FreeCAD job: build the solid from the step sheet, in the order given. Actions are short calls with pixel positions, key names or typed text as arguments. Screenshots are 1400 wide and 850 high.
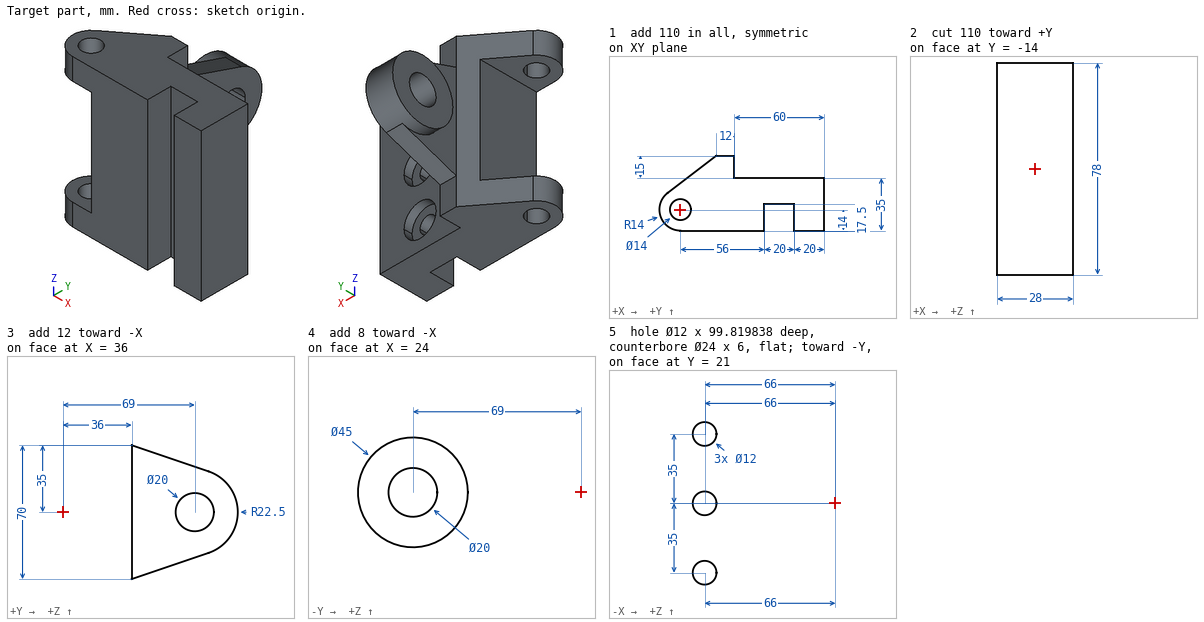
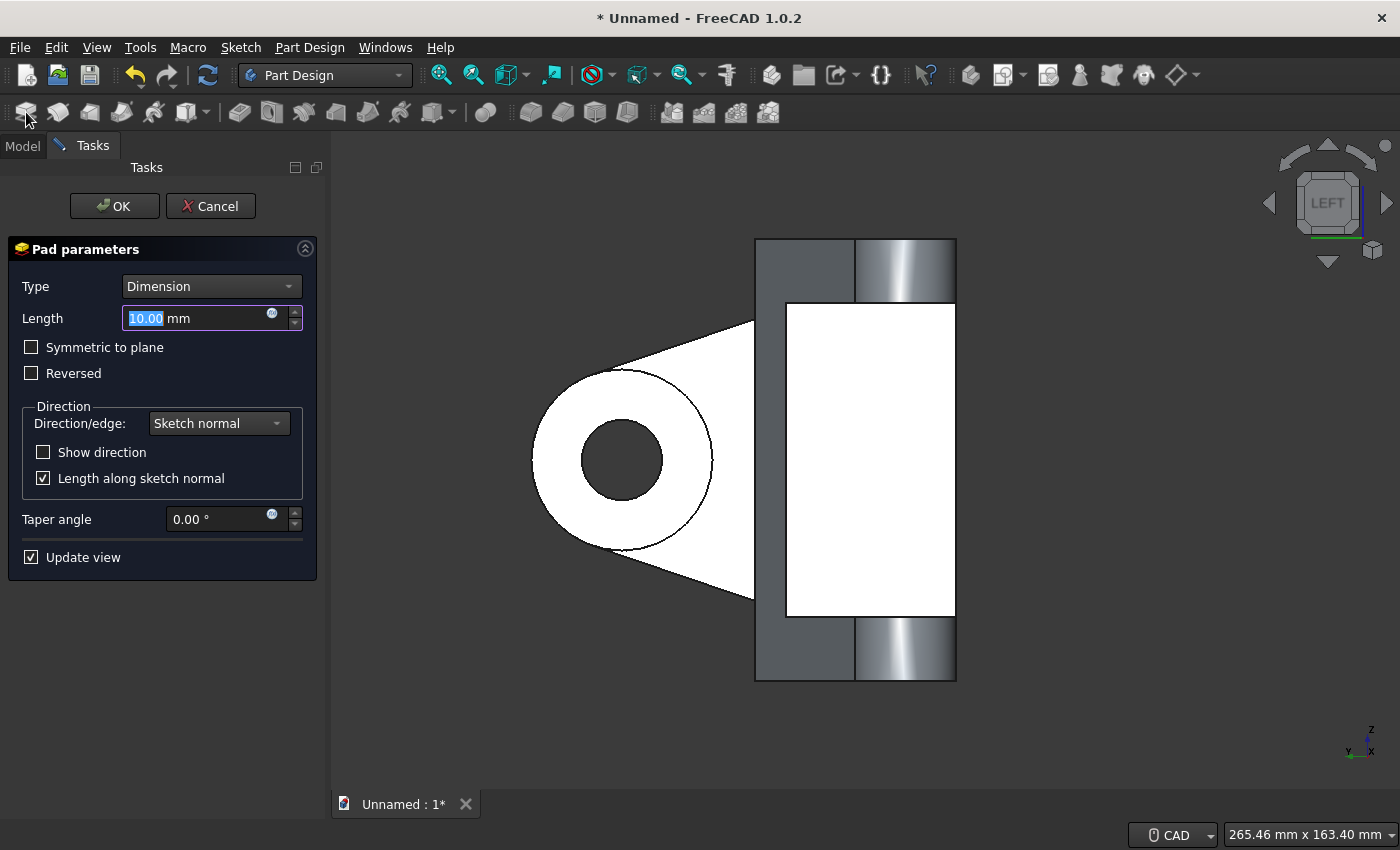
text(8)
key(Tab)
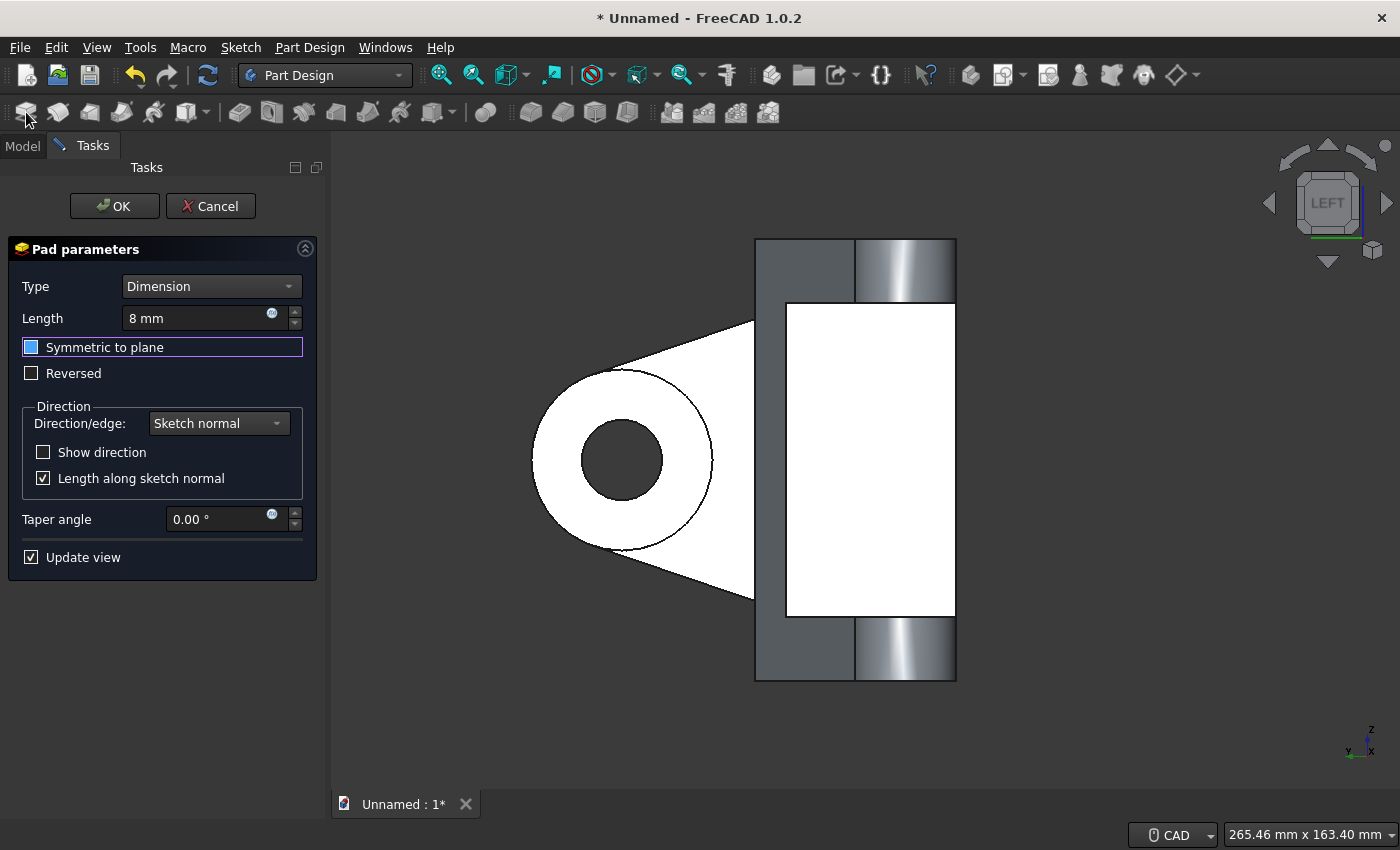
click(115, 206)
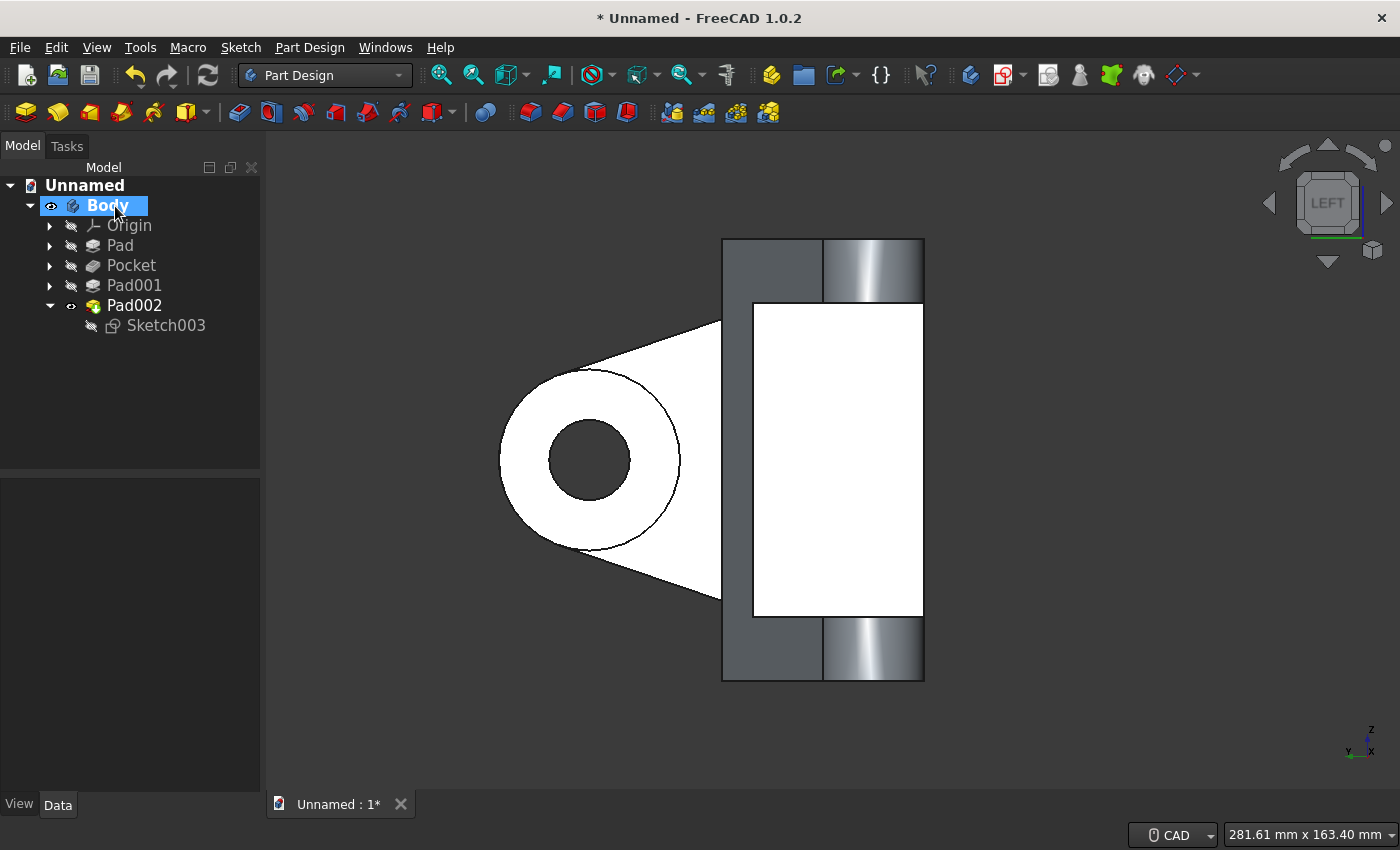
key(4)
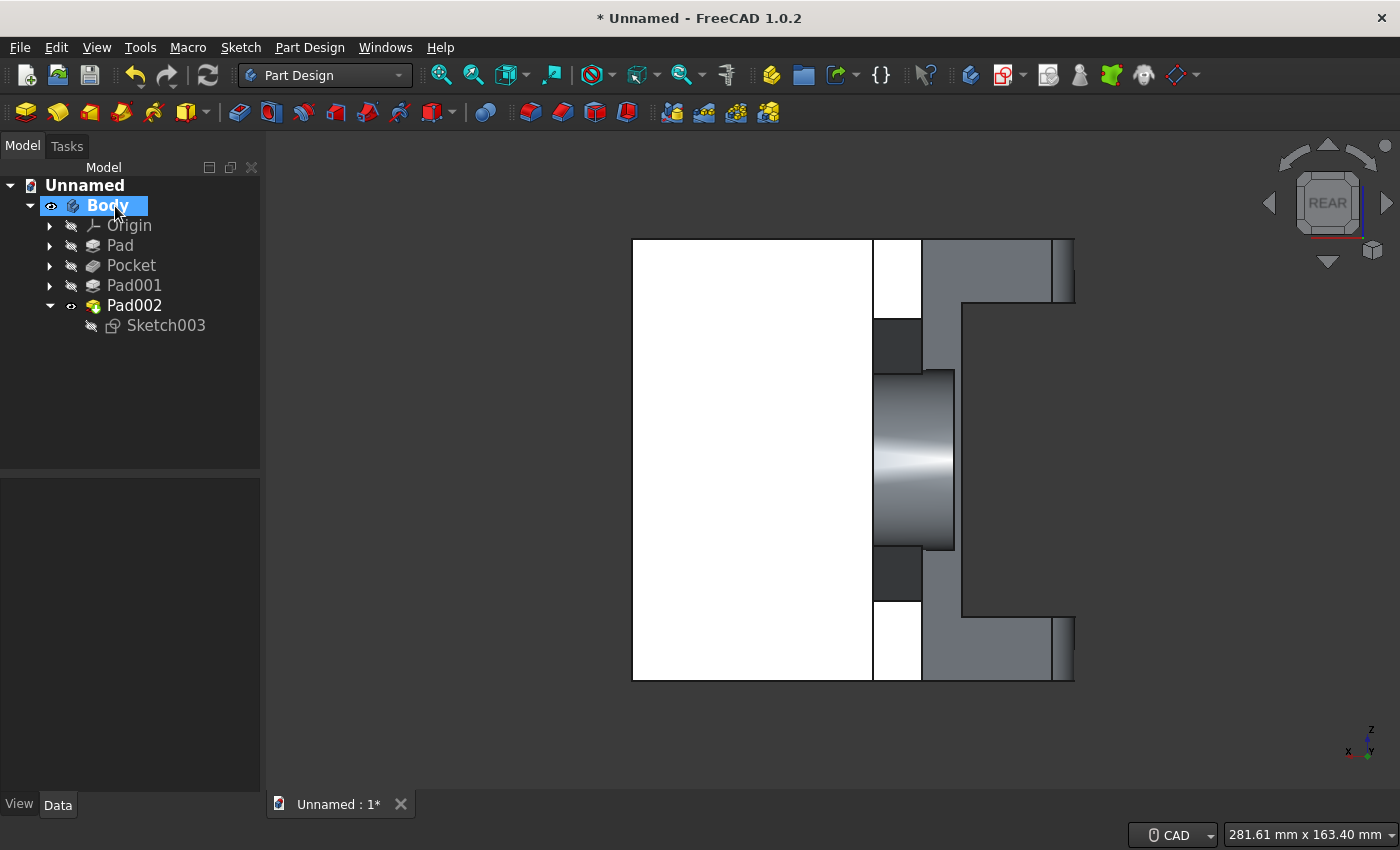
click(752, 396)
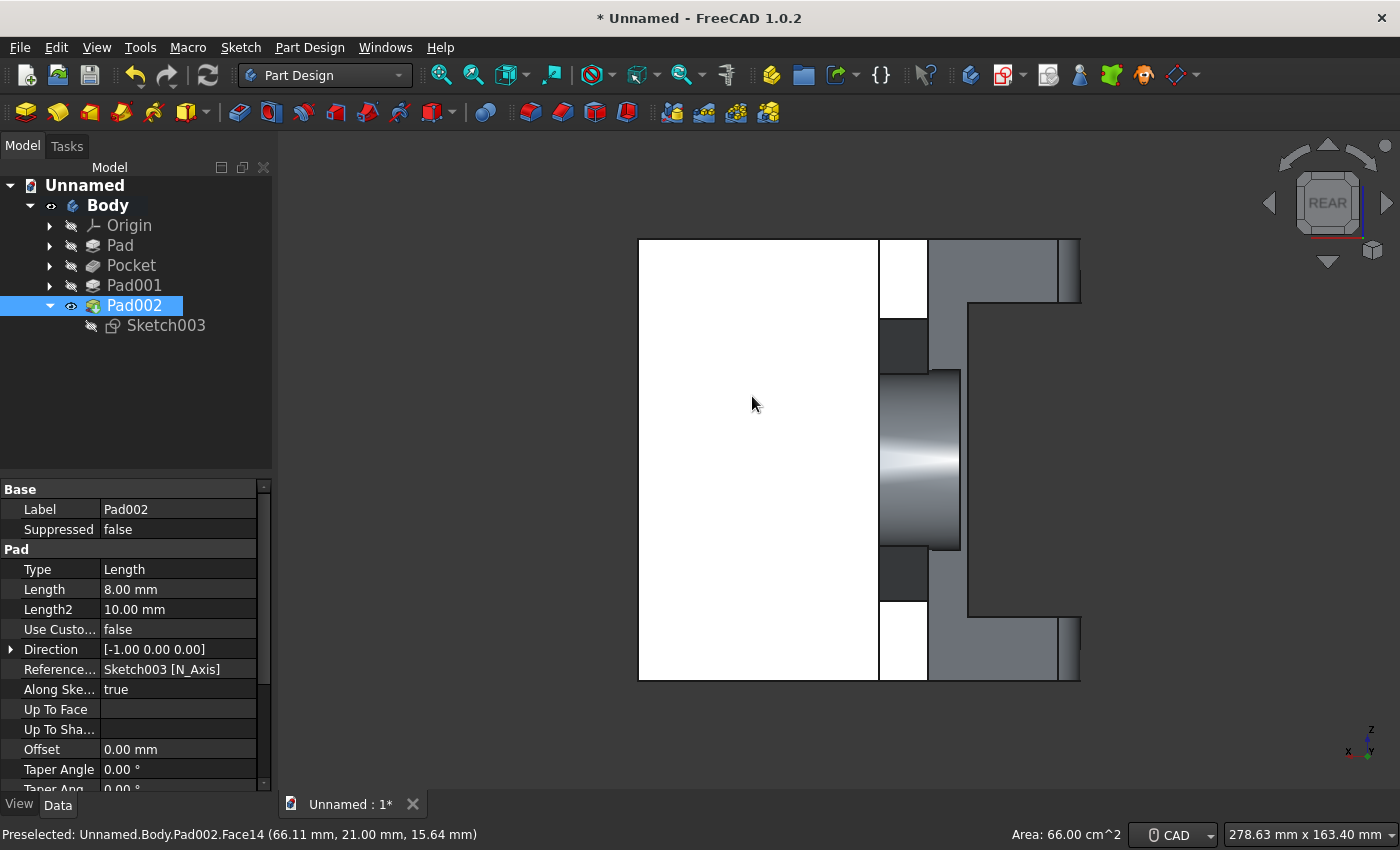
click(1004, 76)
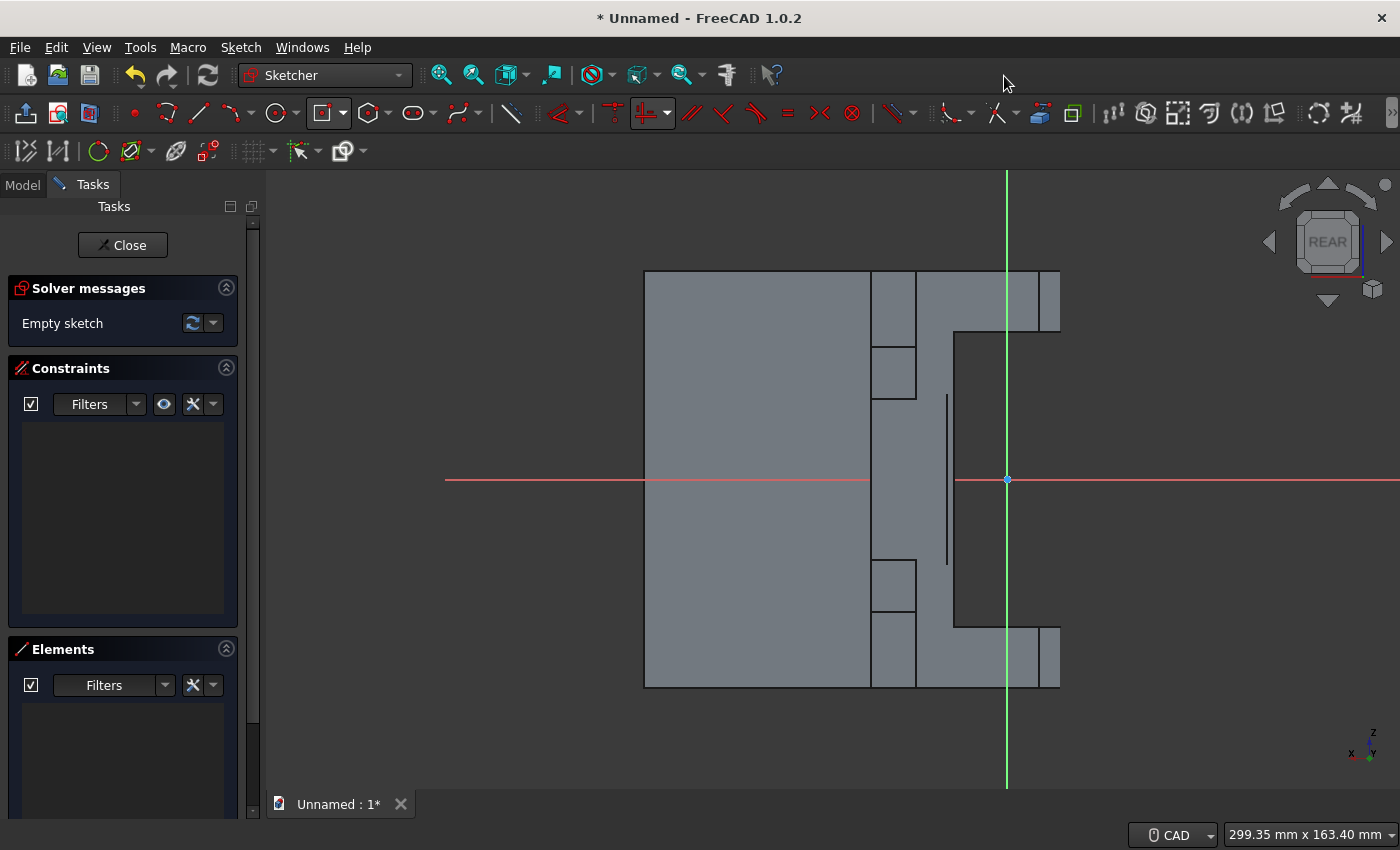
click(90, 114)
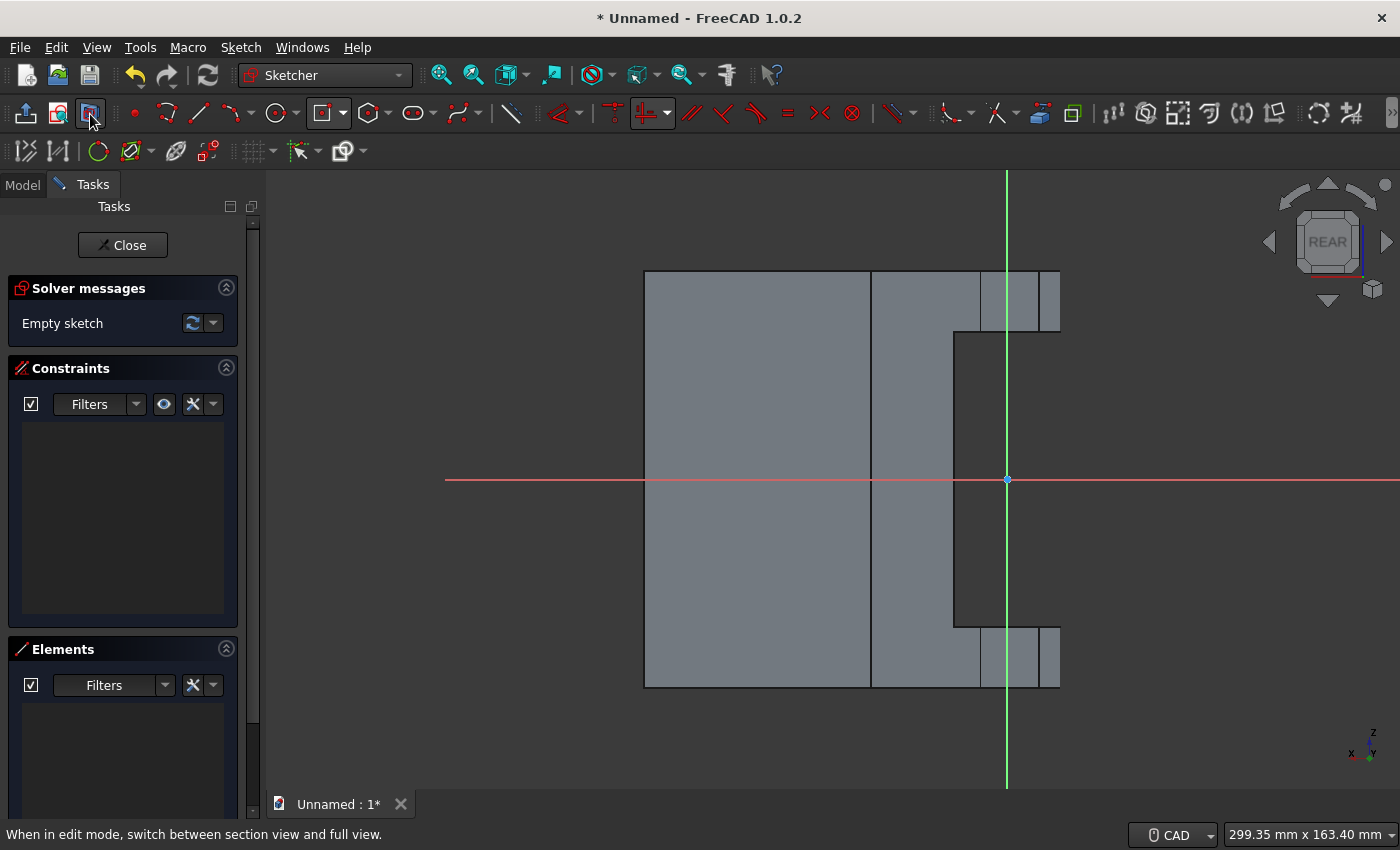
click(276, 114)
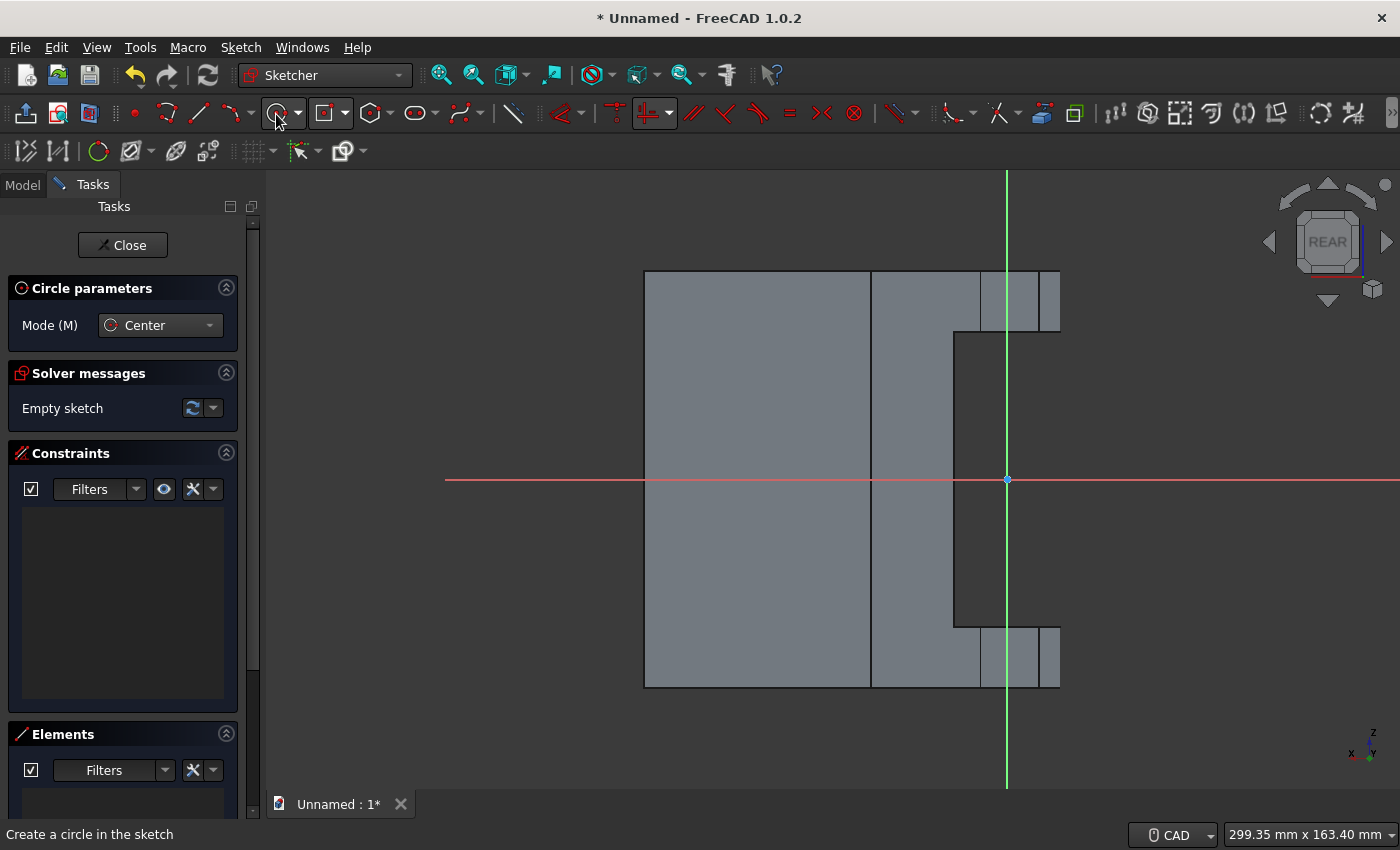
click(757, 347)
click(773, 331)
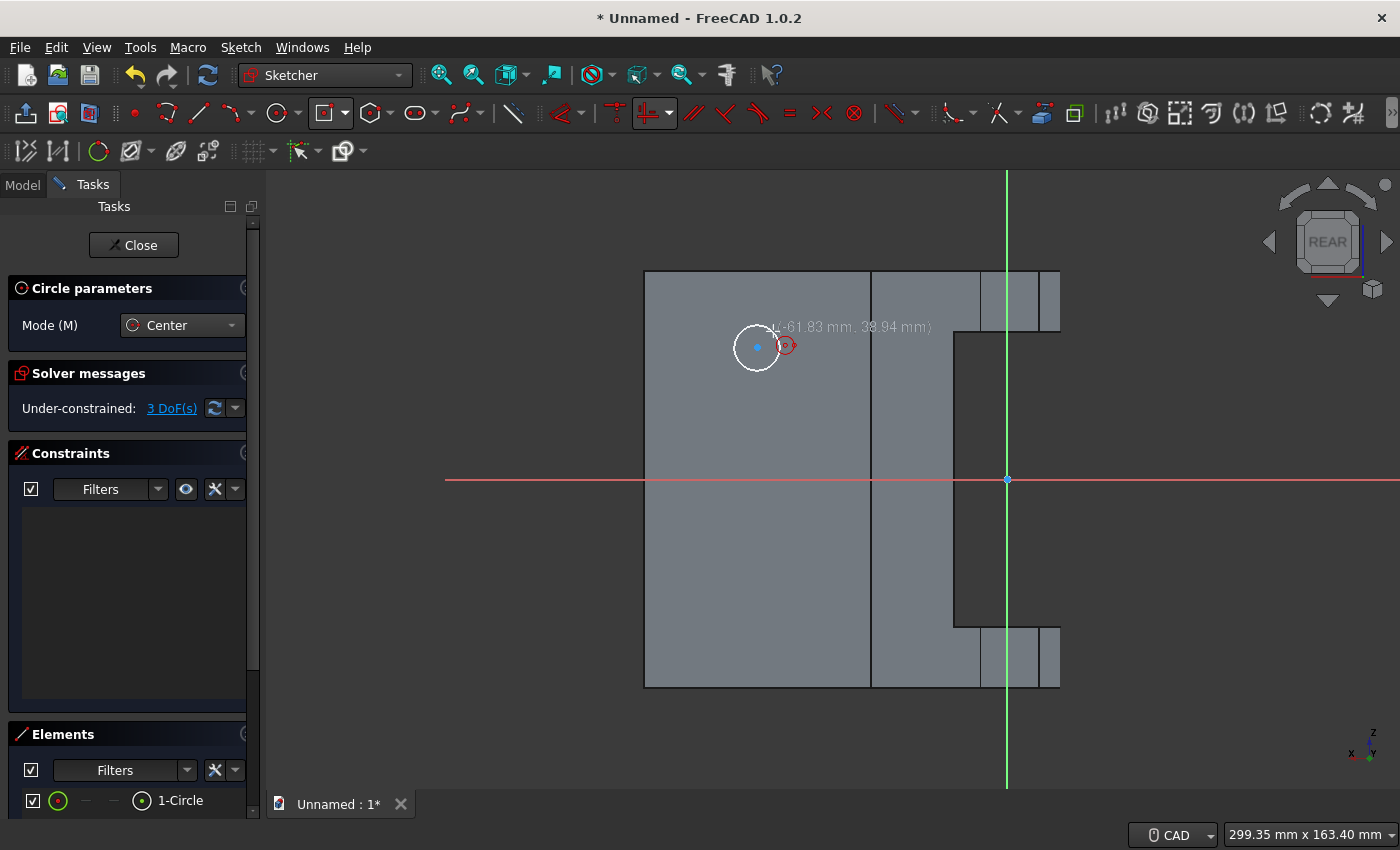
click(757, 480)
click(773, 463)